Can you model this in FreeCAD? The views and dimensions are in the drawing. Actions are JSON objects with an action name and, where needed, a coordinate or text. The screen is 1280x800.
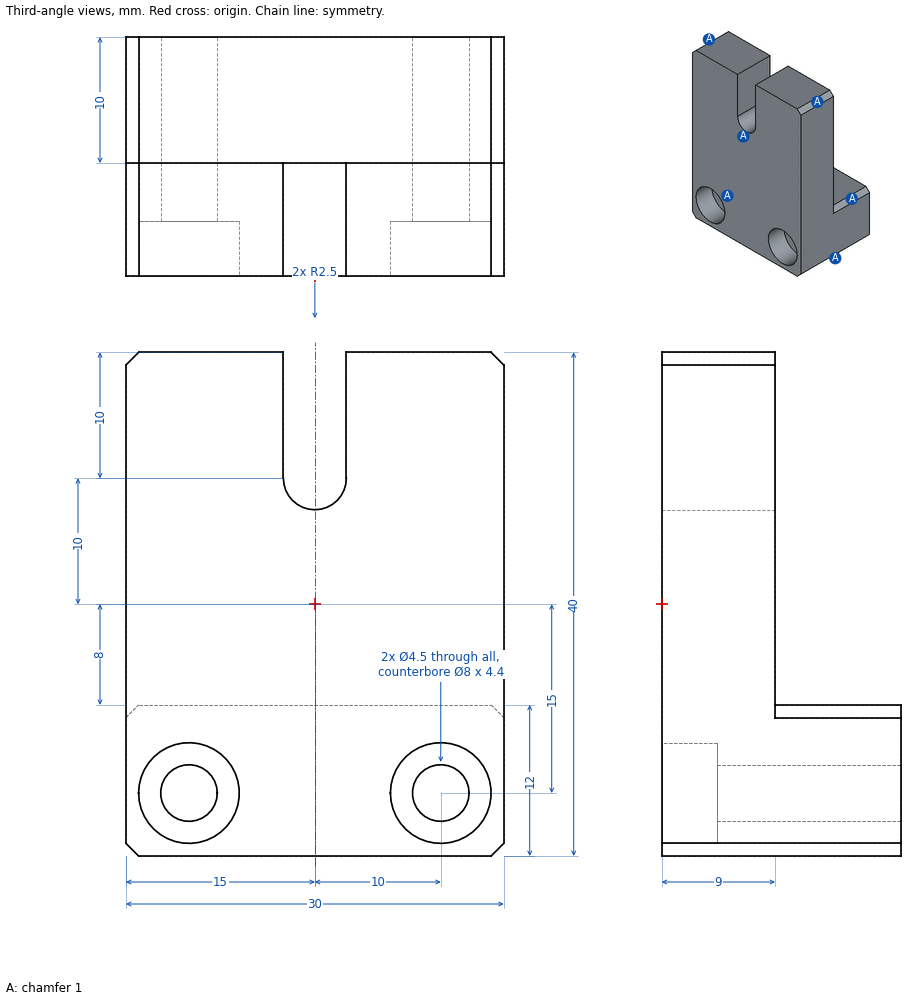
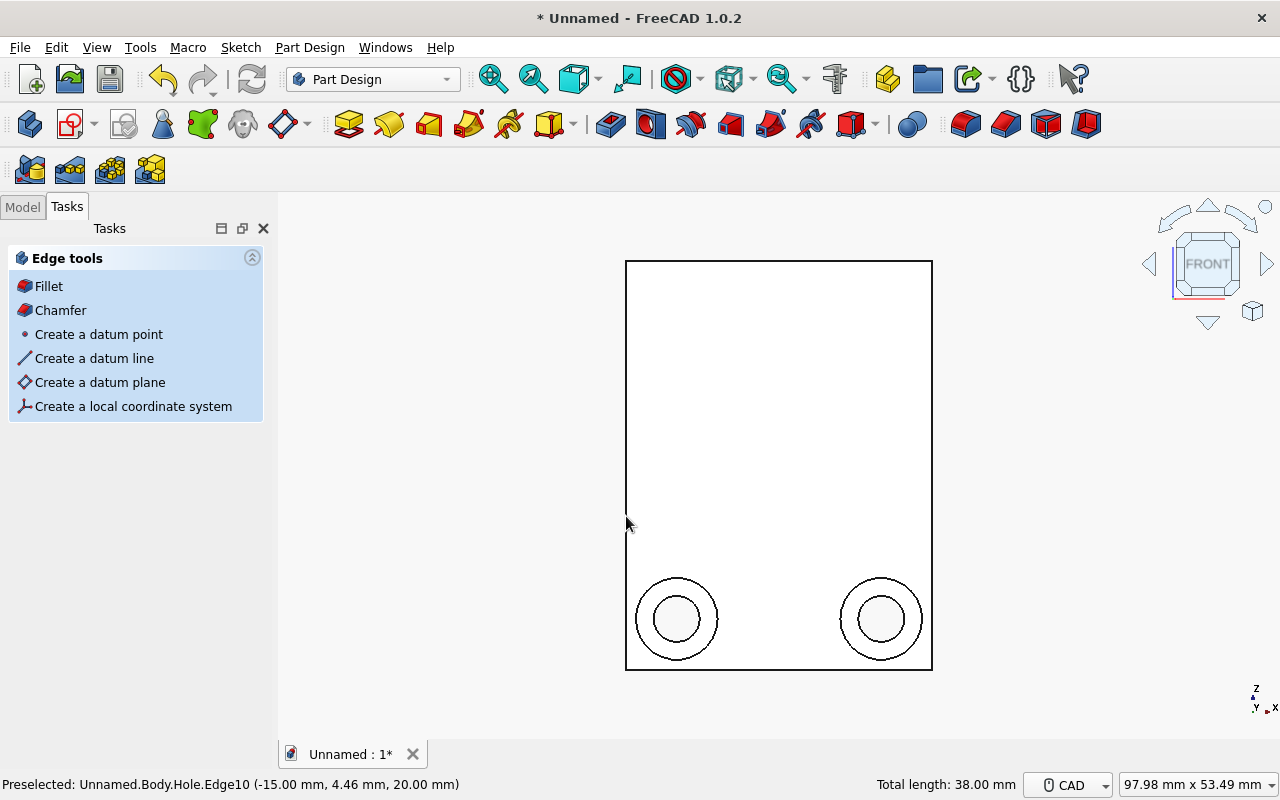
{"action": "key", "text": "3"}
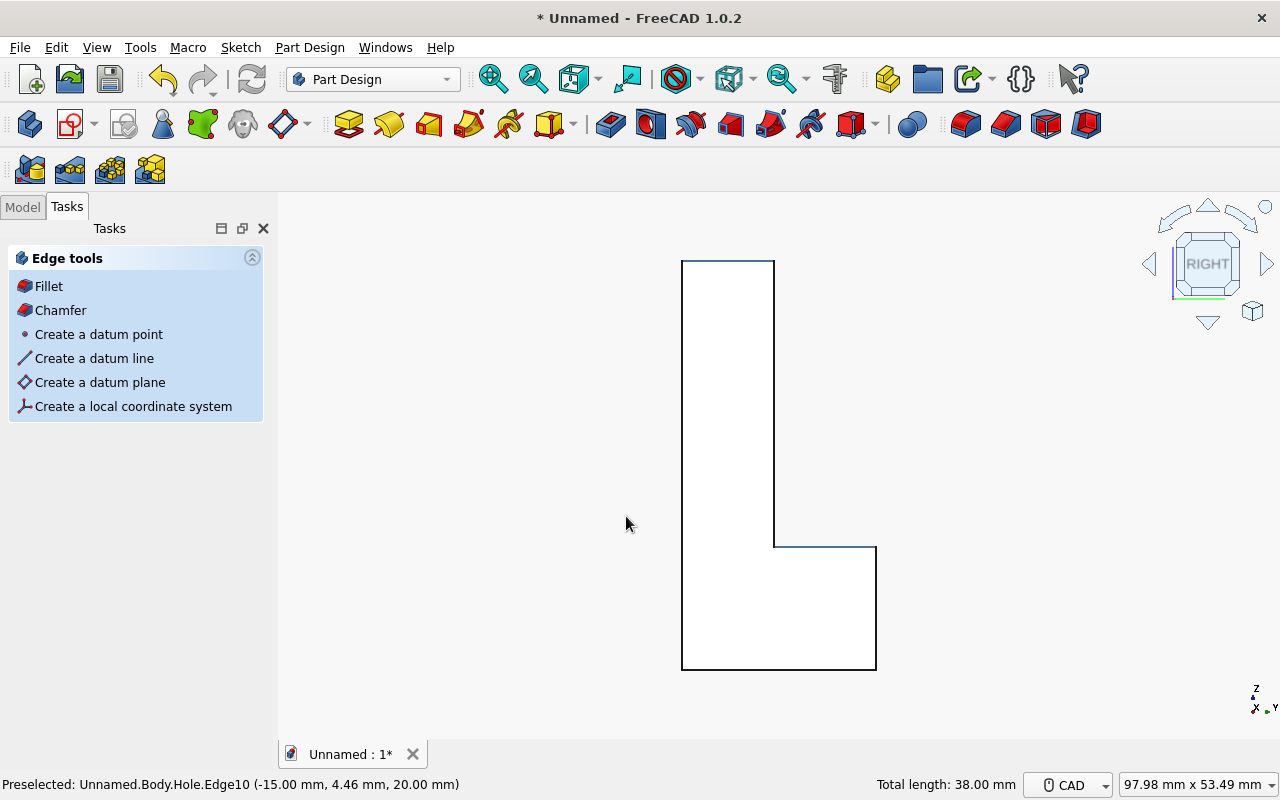
{"action": "left_click", "coordinate": [779, 669], "text": "ctrl"}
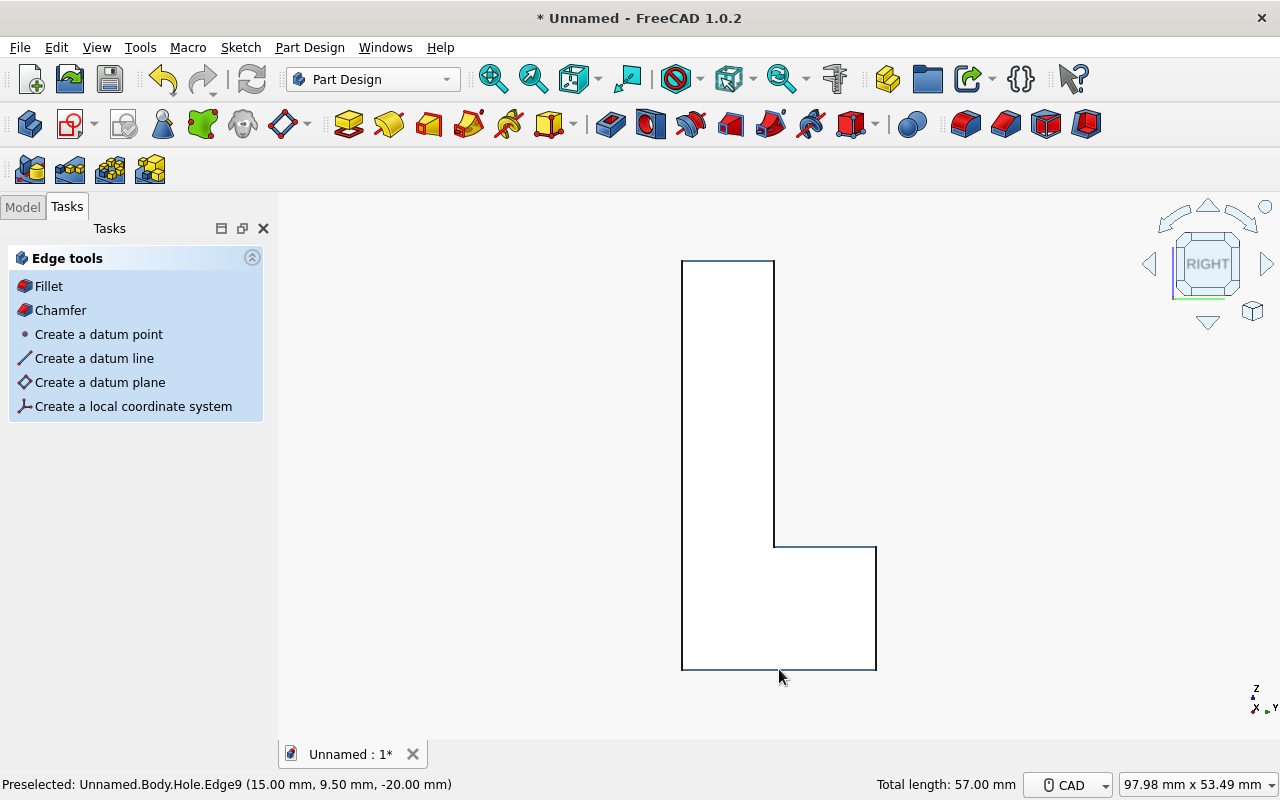
{"action": "key", "text": "5"}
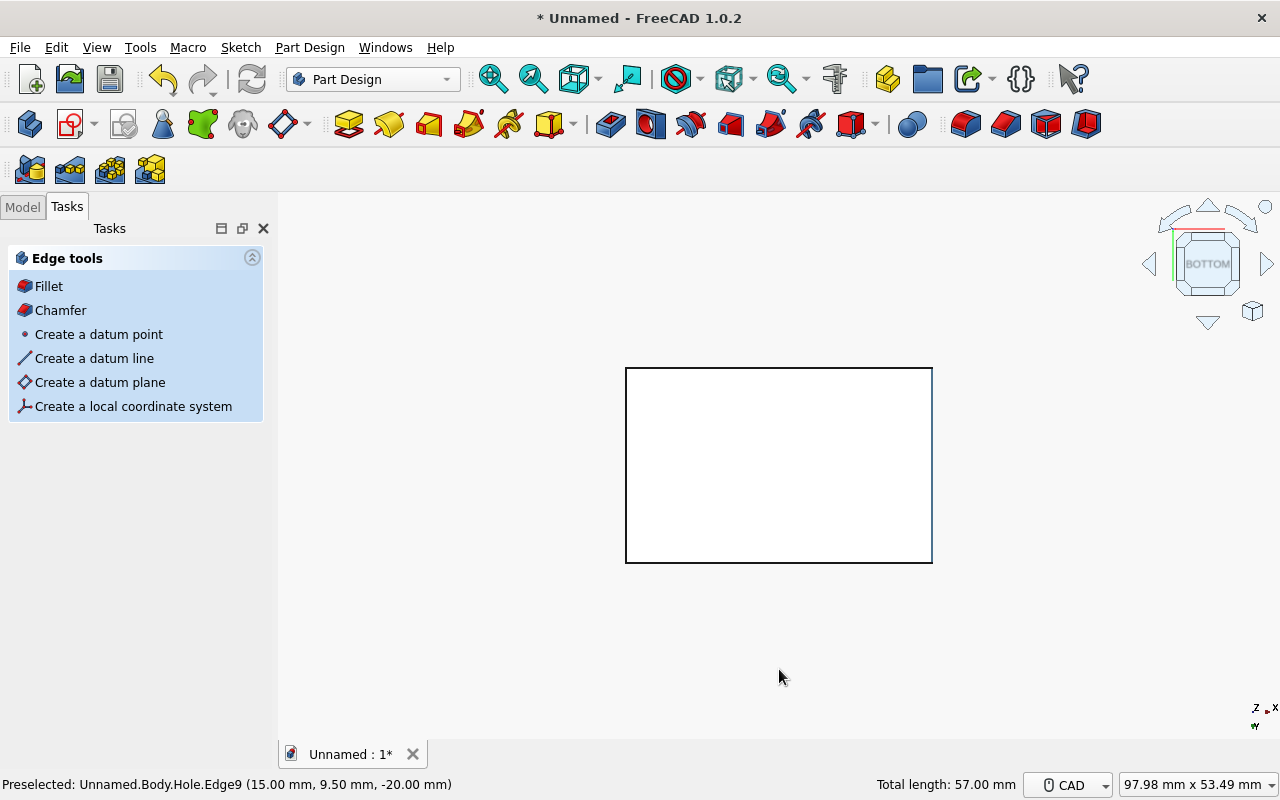
{"action": "left_click", "coordinate": [494, 80]}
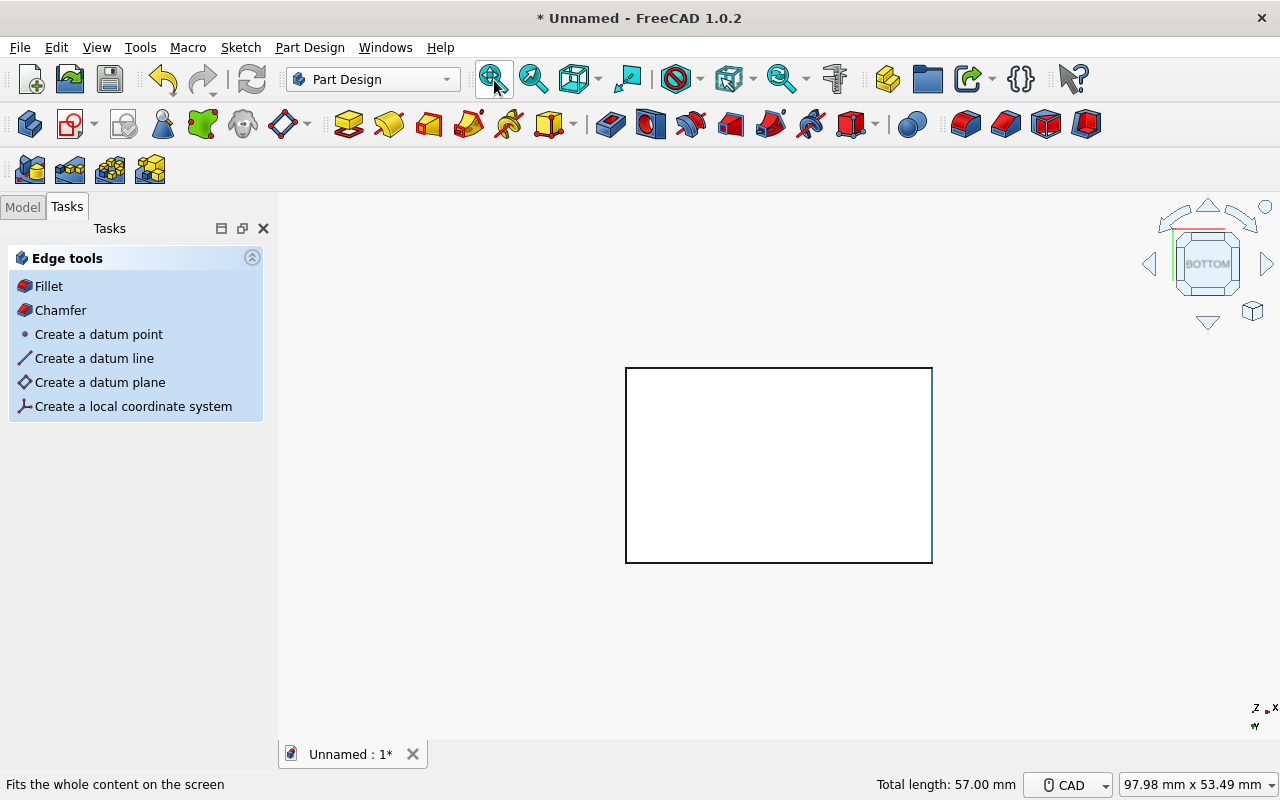
{"action": "left_click", "coordinate": [626, 464], "text": "ctrl"}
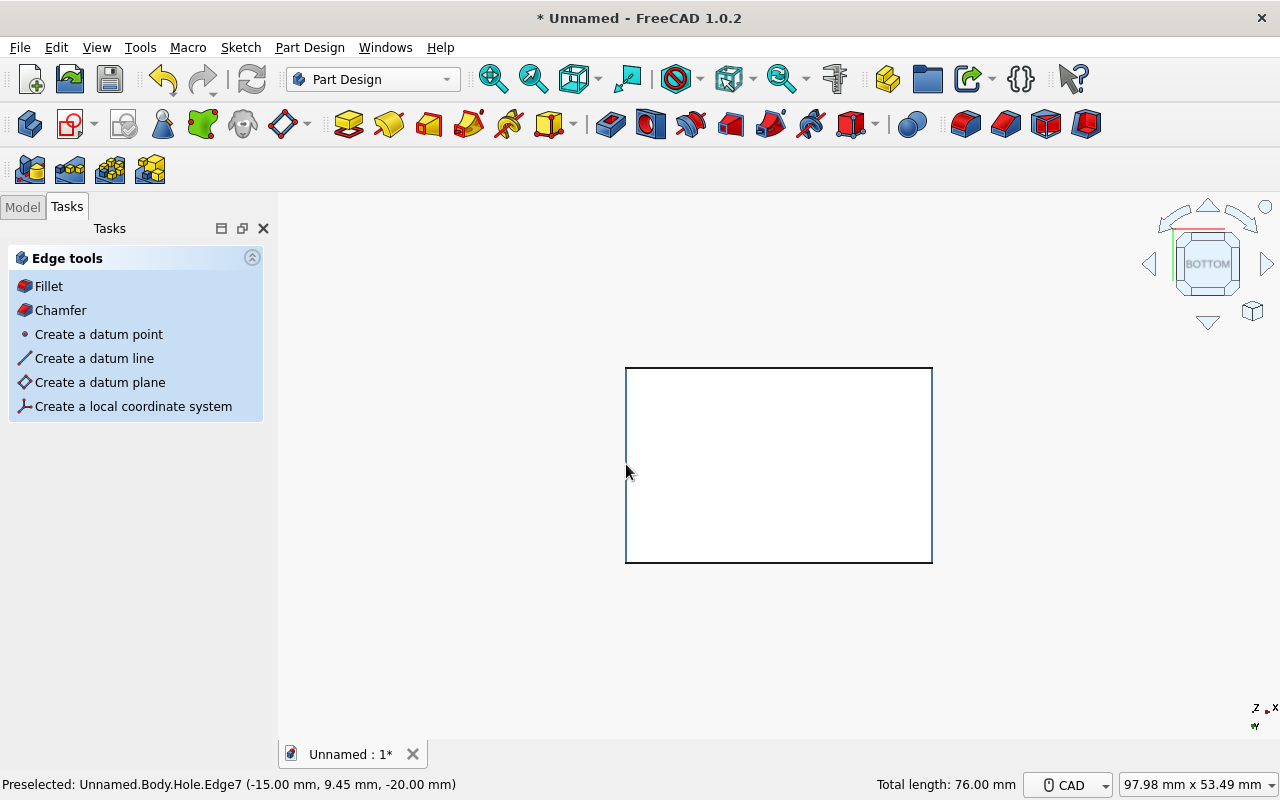
{"action": "left_click", "coordinate": [1006, 124]}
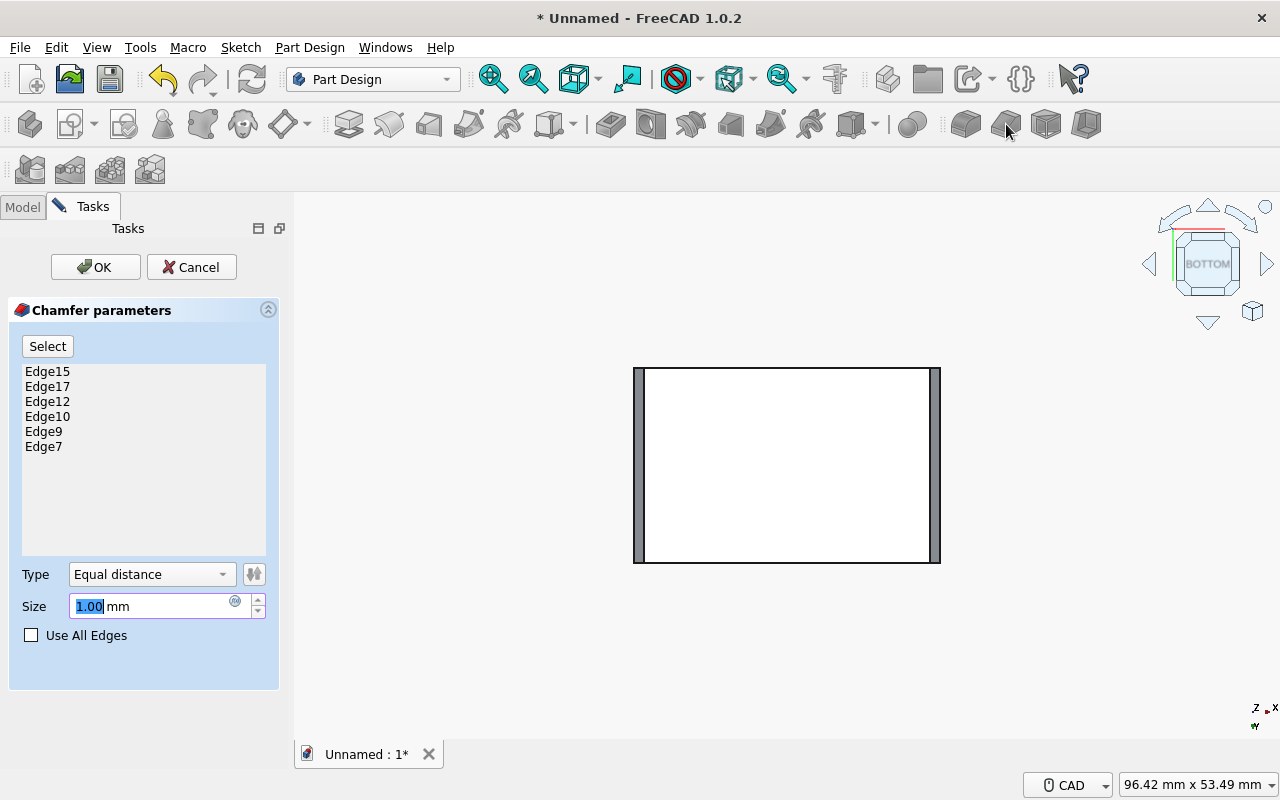
{"action": "type", "text": "1"}
{"action": "key", "text": "Tab"}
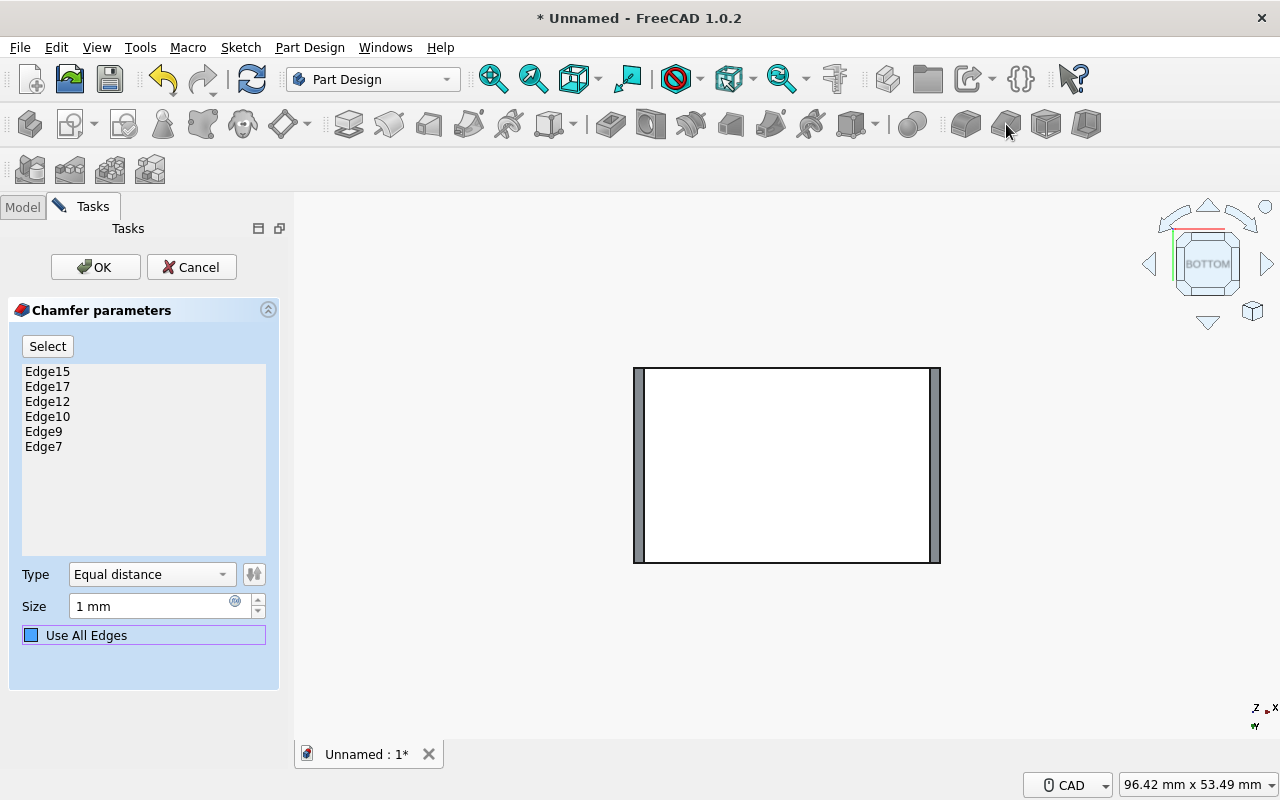
{"action": "left_click", "coordinate": [96, 267]}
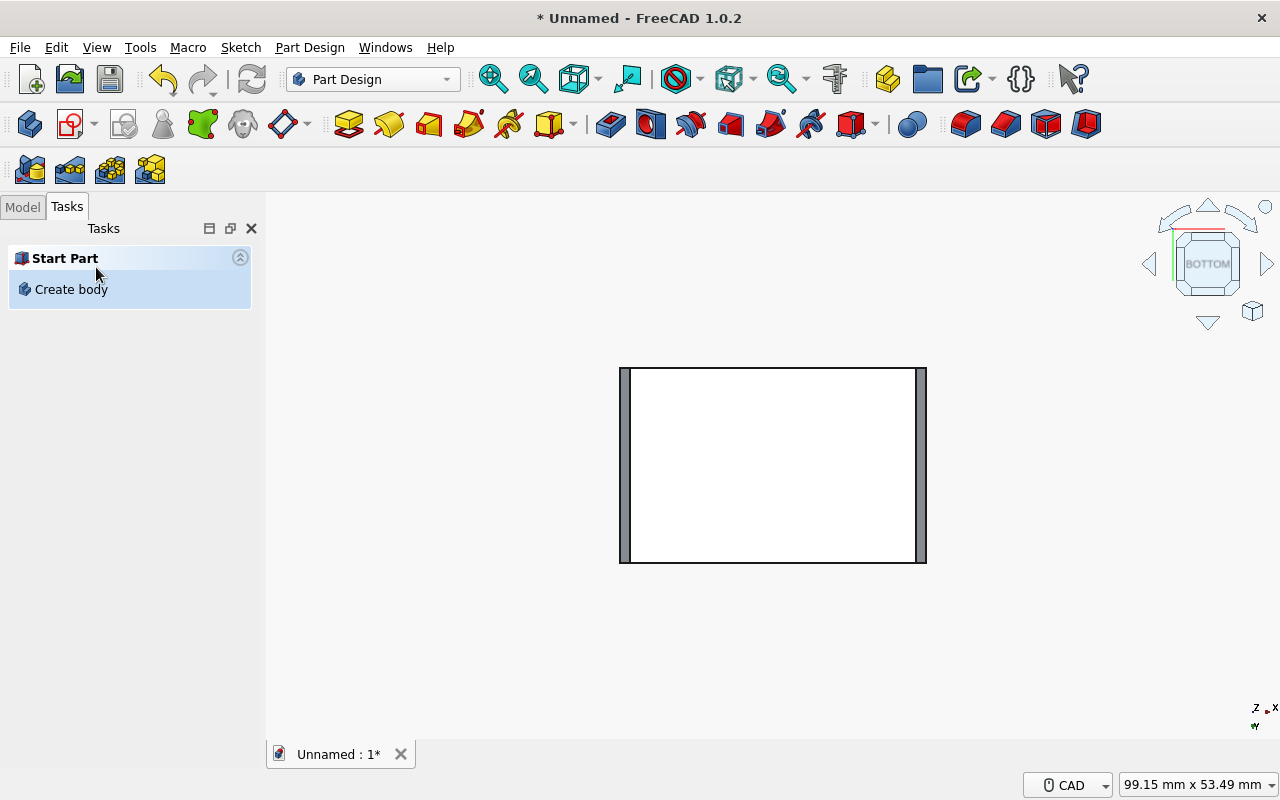
{"action": "left_click", "coordinate": [494, 80]}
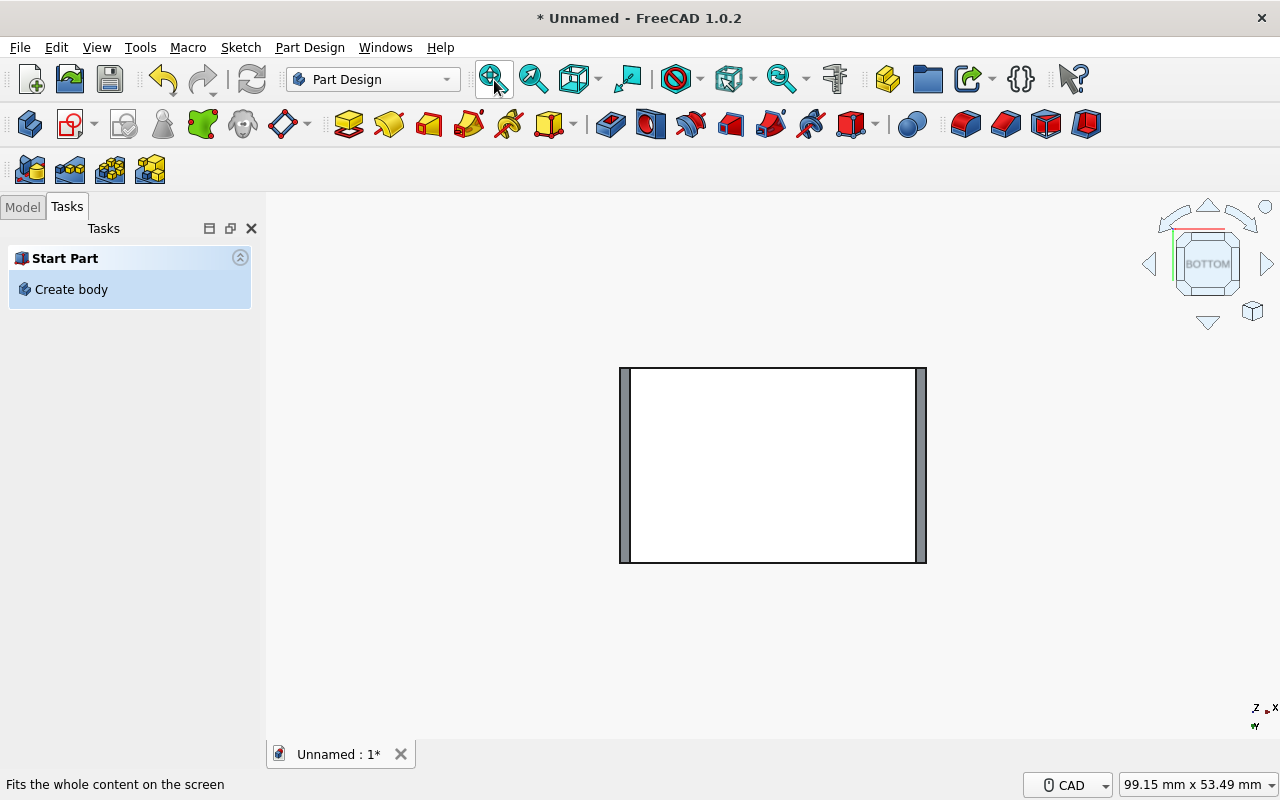
{"action": "key", "text": "0"}